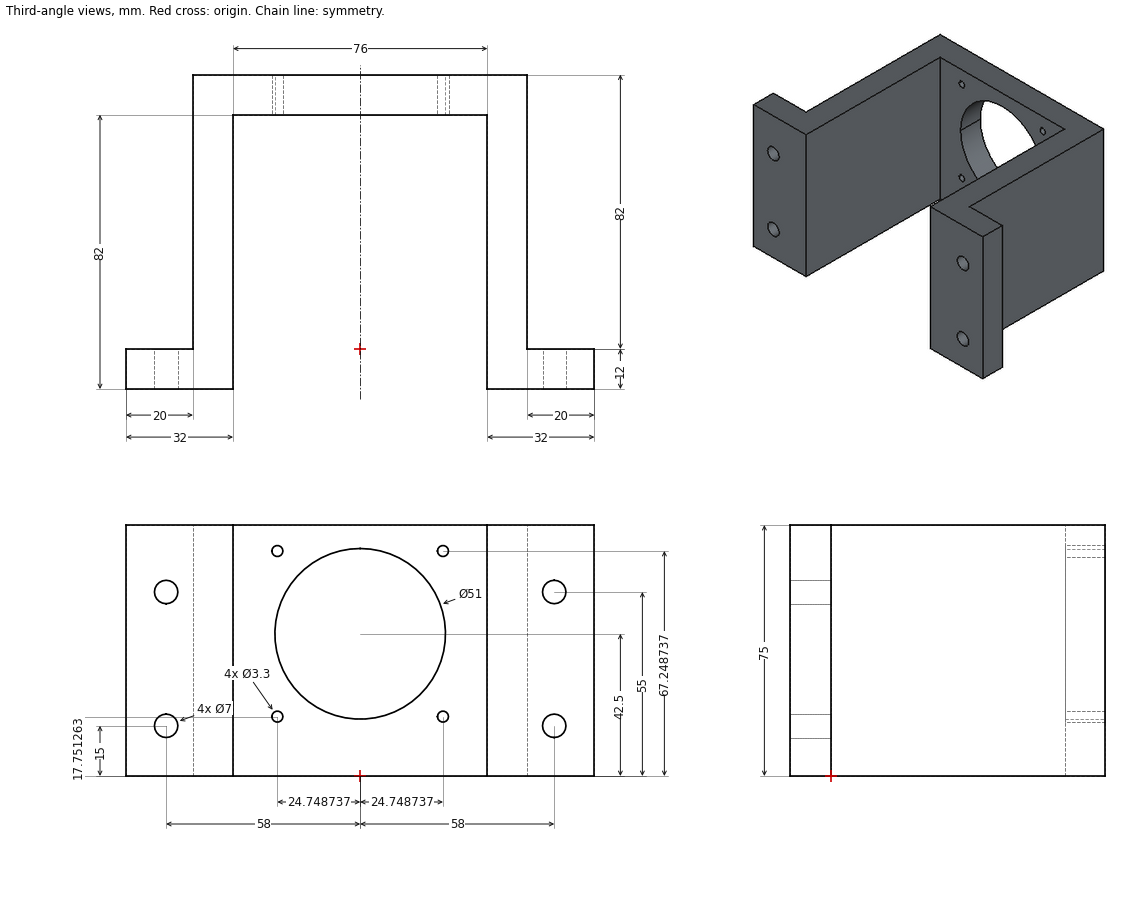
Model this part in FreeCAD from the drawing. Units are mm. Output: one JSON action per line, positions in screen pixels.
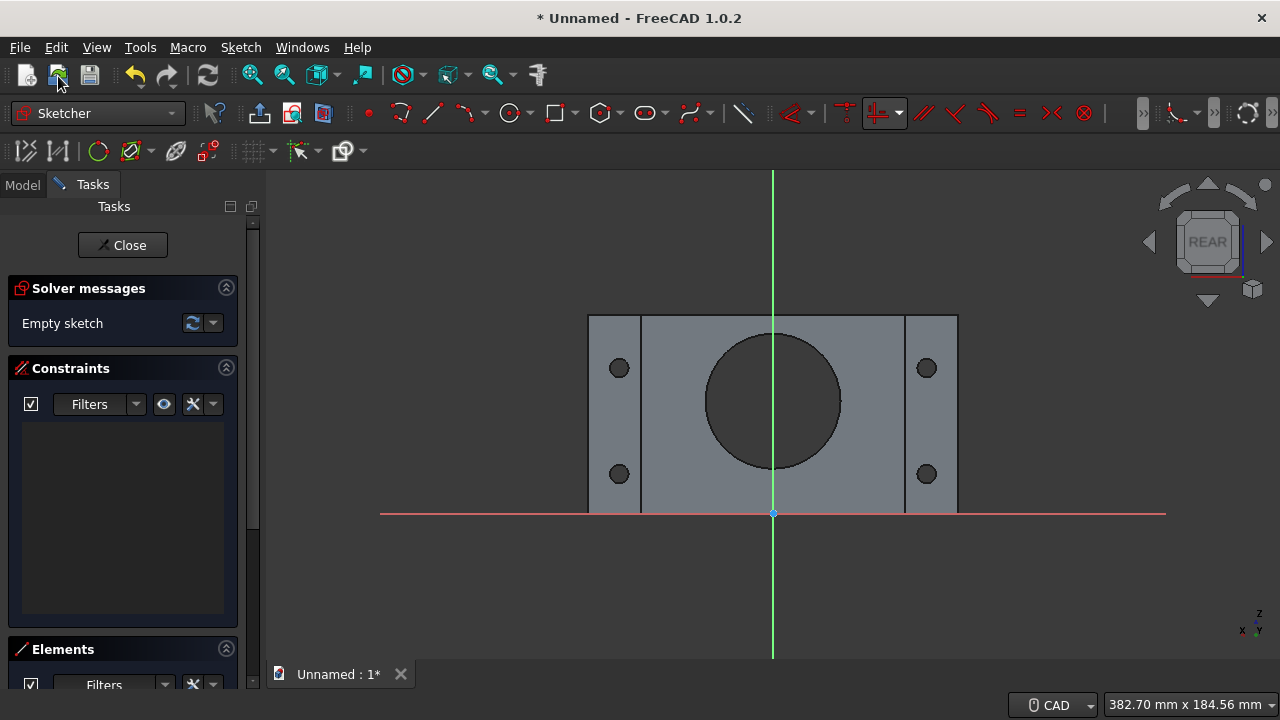
{"action": "scroll", "coordinate": [856, 432], "scroll_direction": "up", "scroll_amount": 3}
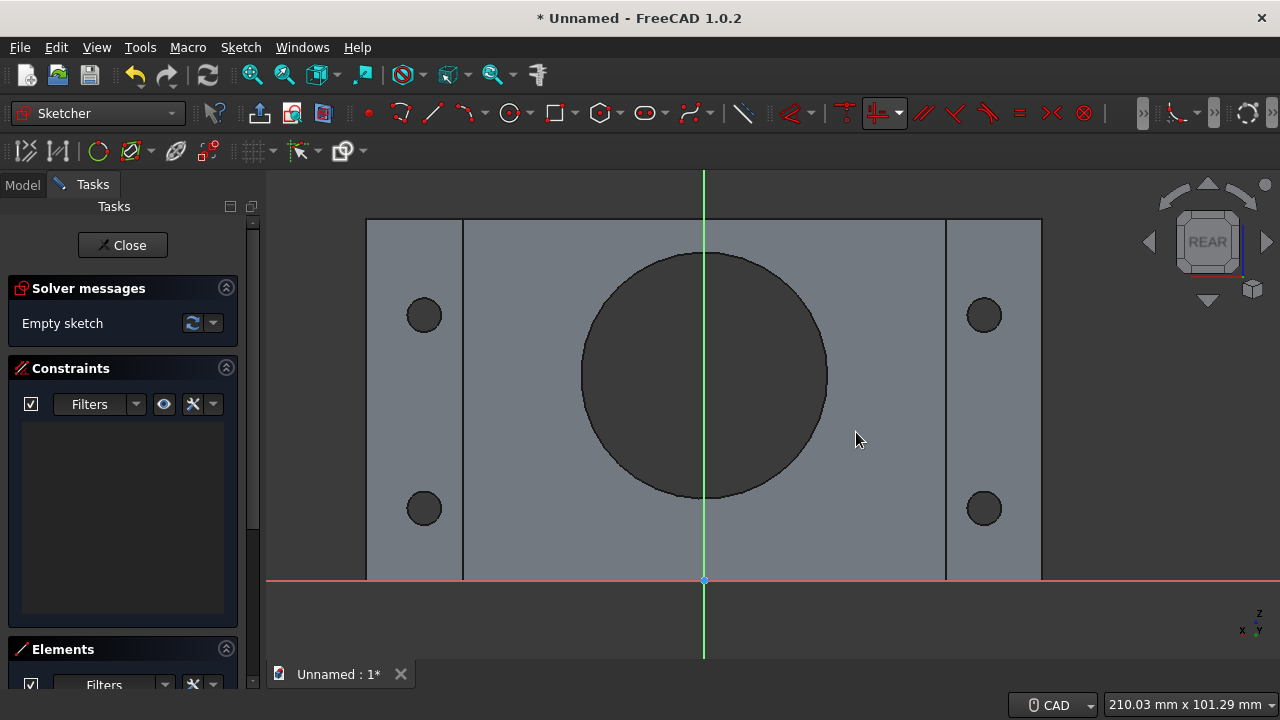
{"action": "left_click", "coordinate": [510, 114]}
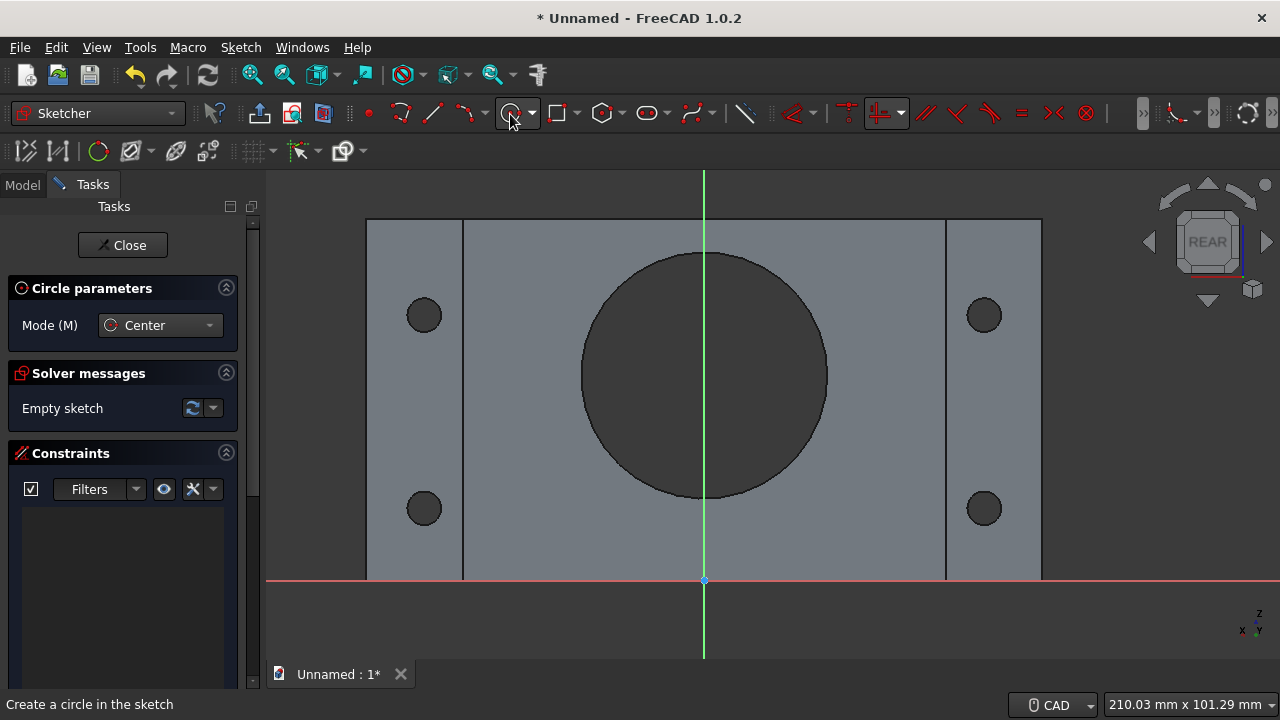
{"action": "scroll", "coordinate": [824, 495], "scroll_direction": "up", "scroll_amount": 6}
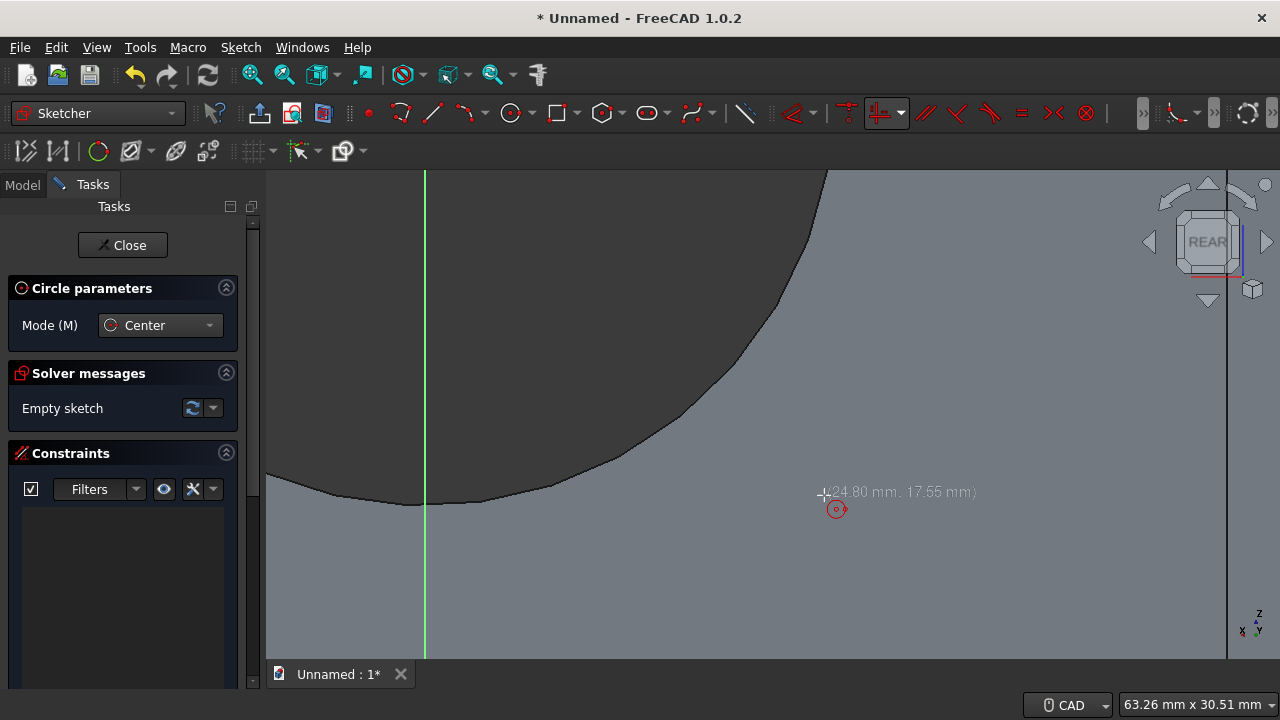
{"action": "left_click", "coordinate": [822, 494]}
{"action": "mouse_move", "coordinate": [841, 475]}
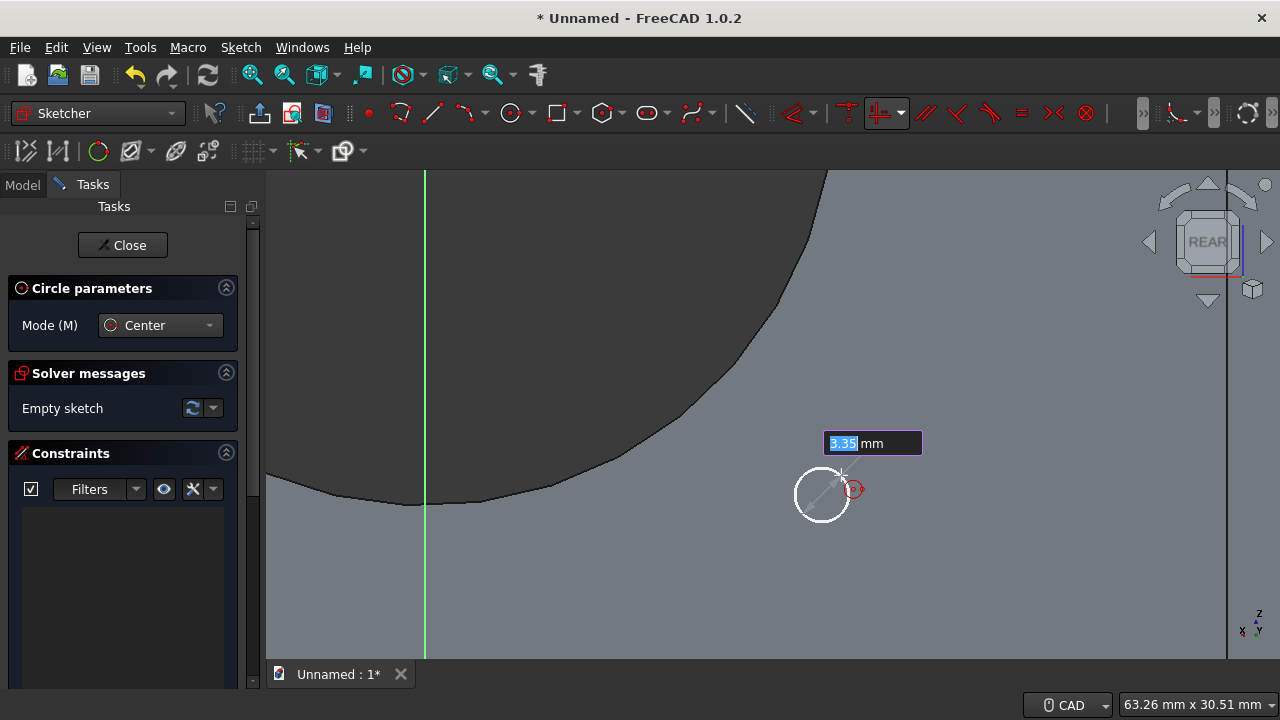
{"action": "type", "text": "3.3"}
{"action": "key", "text": "Return"}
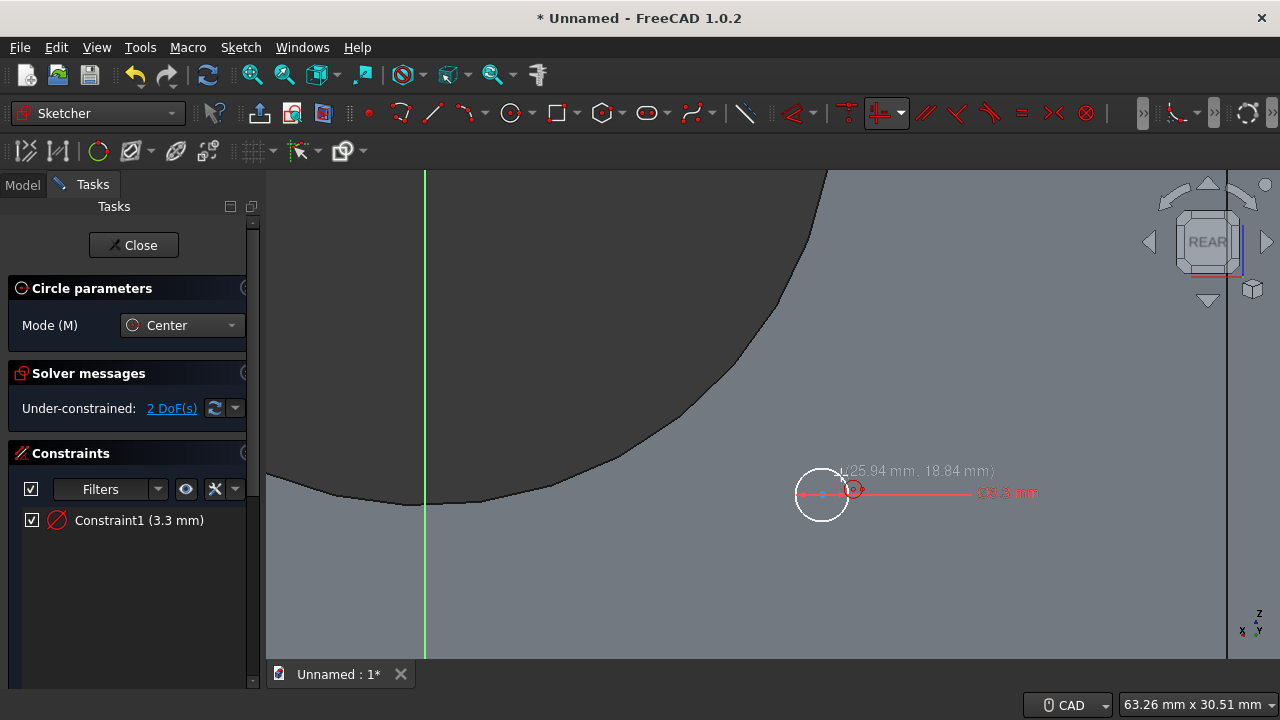
{"action": "scroll", "coordinate": [825, 496], "scroll_direction": "down", "scroll_amount": 6}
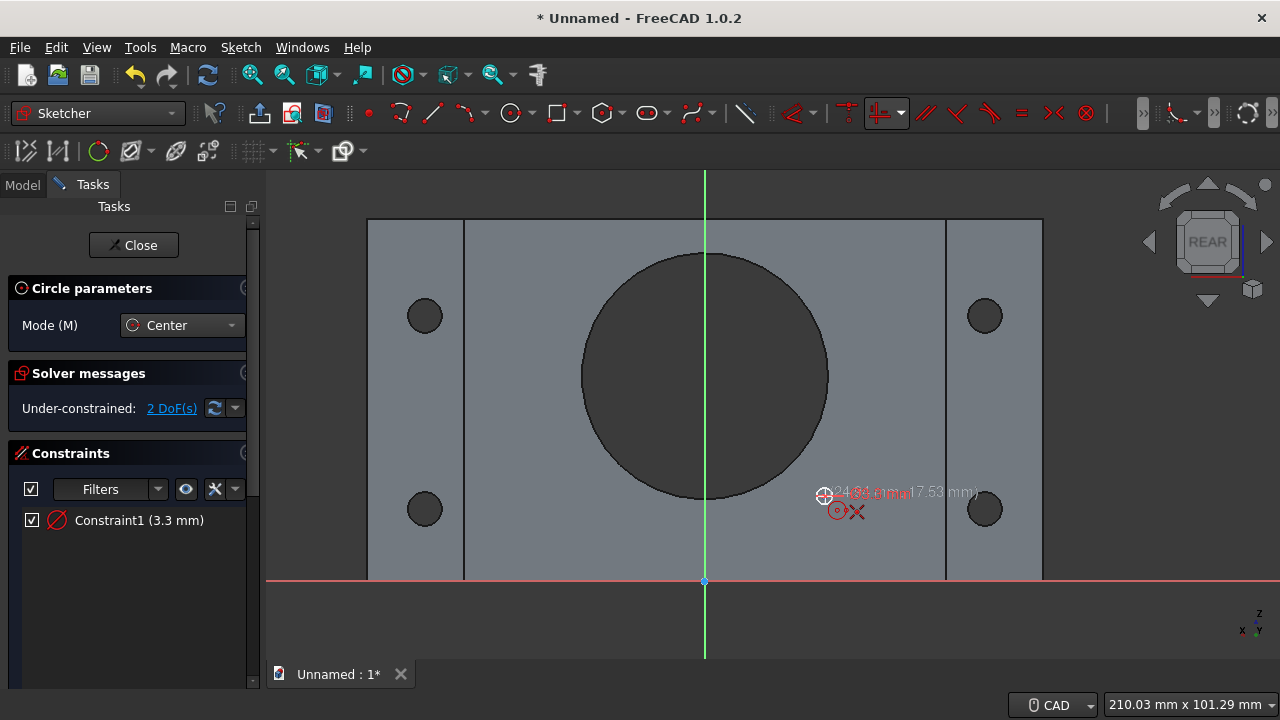
{"action": "scroll", "coordinate": [586, 496], "scroll_direction": "up", "scroll_amount": 6}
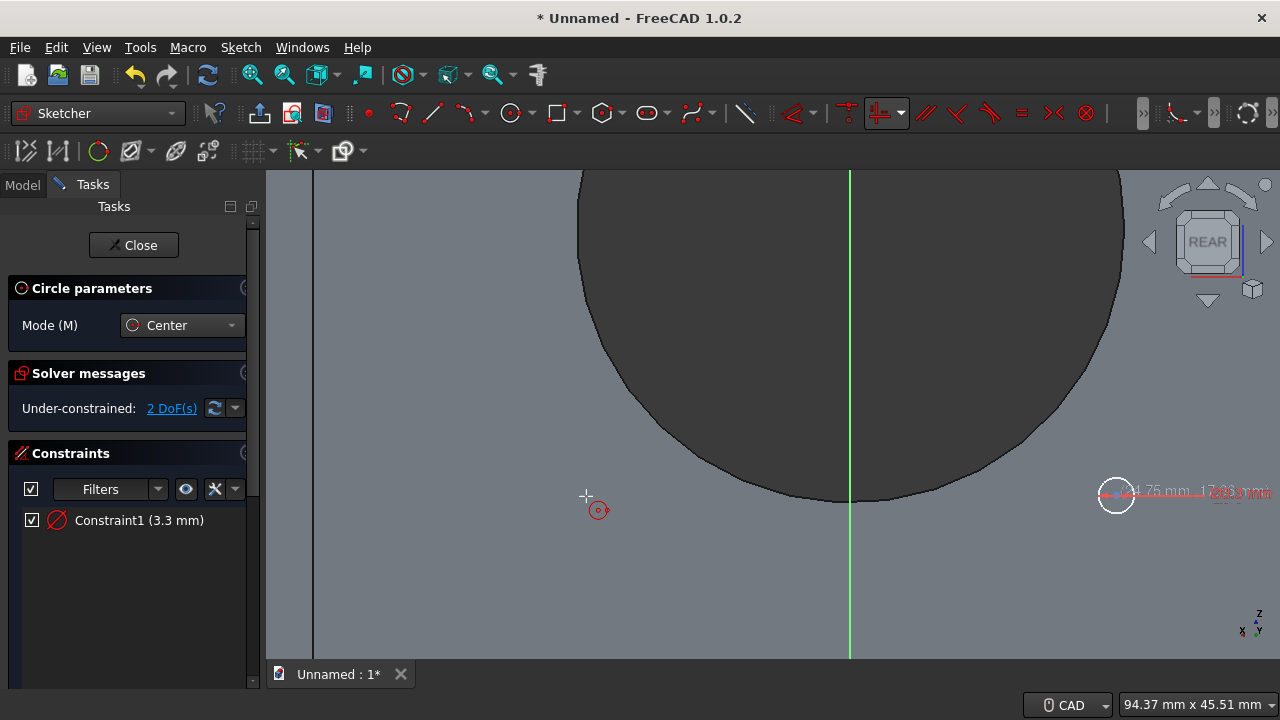
{"action": "left_click", "coordinate": [584, 494]}
{"action": "mouse_move", "coordinate": [602, 475]}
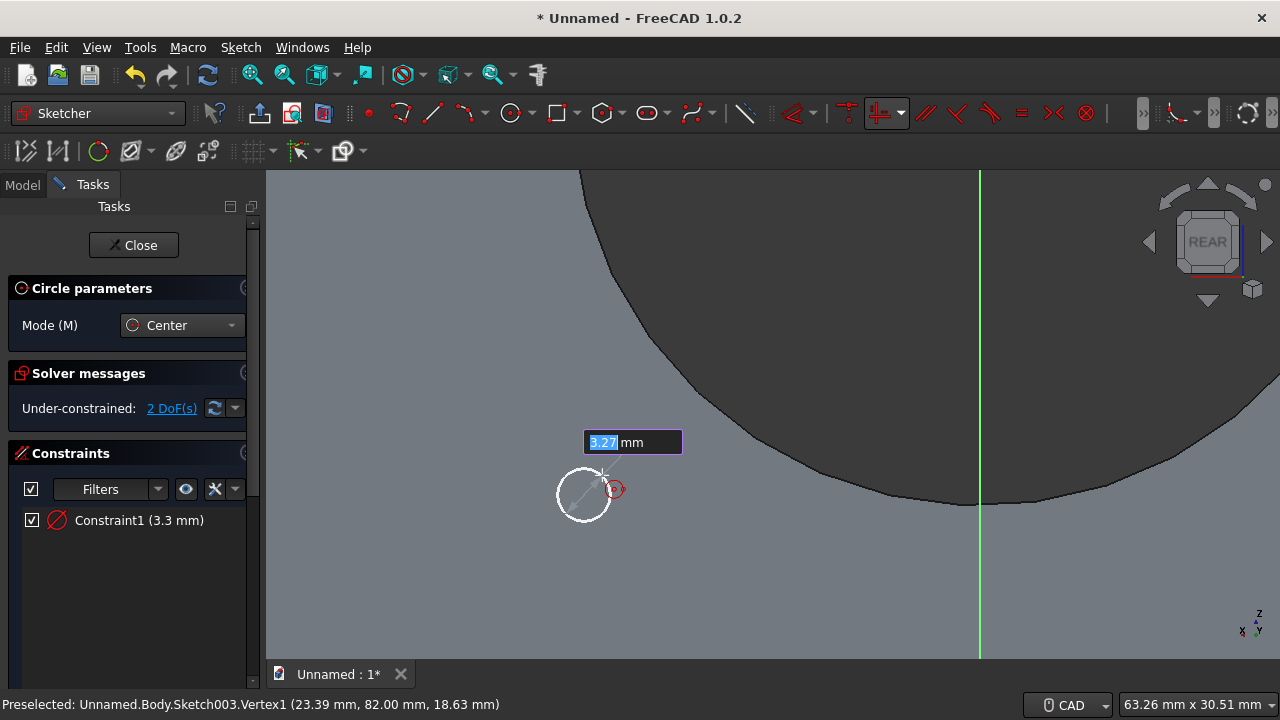
{"action": "type", "text": "3.3"}
{"action": "key", "text": "Return"}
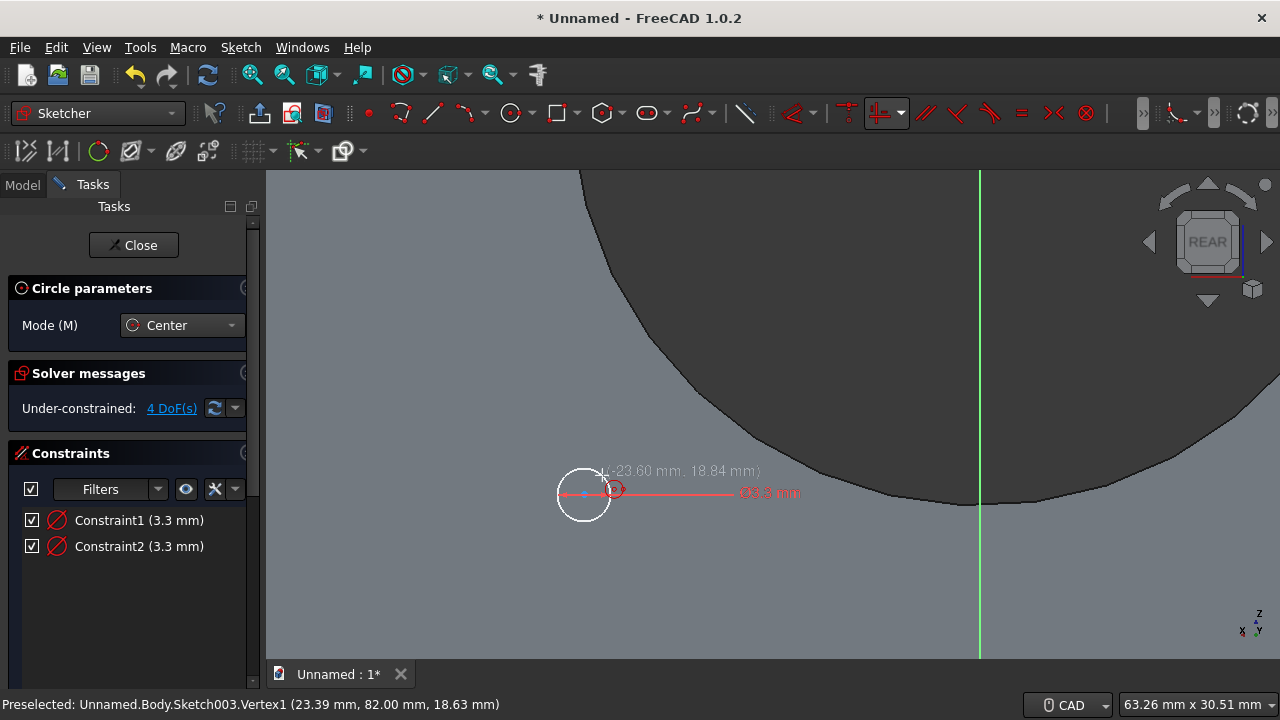
{"action": "scroll", "coordinate": [586, 496], "scroll_direction": "down", "scroll_amount": 6}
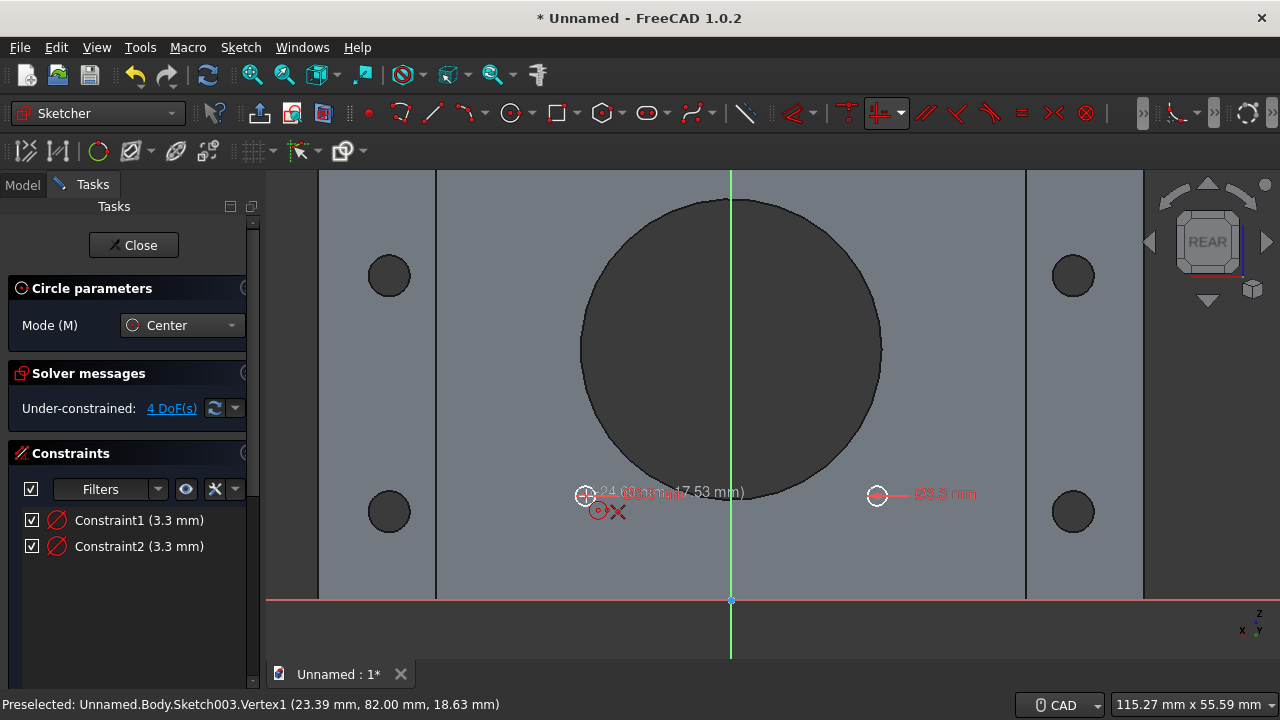
{"action": "scroll", "coordinate": [586, 257], "scroll_direction": "up", "scroll_amount": 6}